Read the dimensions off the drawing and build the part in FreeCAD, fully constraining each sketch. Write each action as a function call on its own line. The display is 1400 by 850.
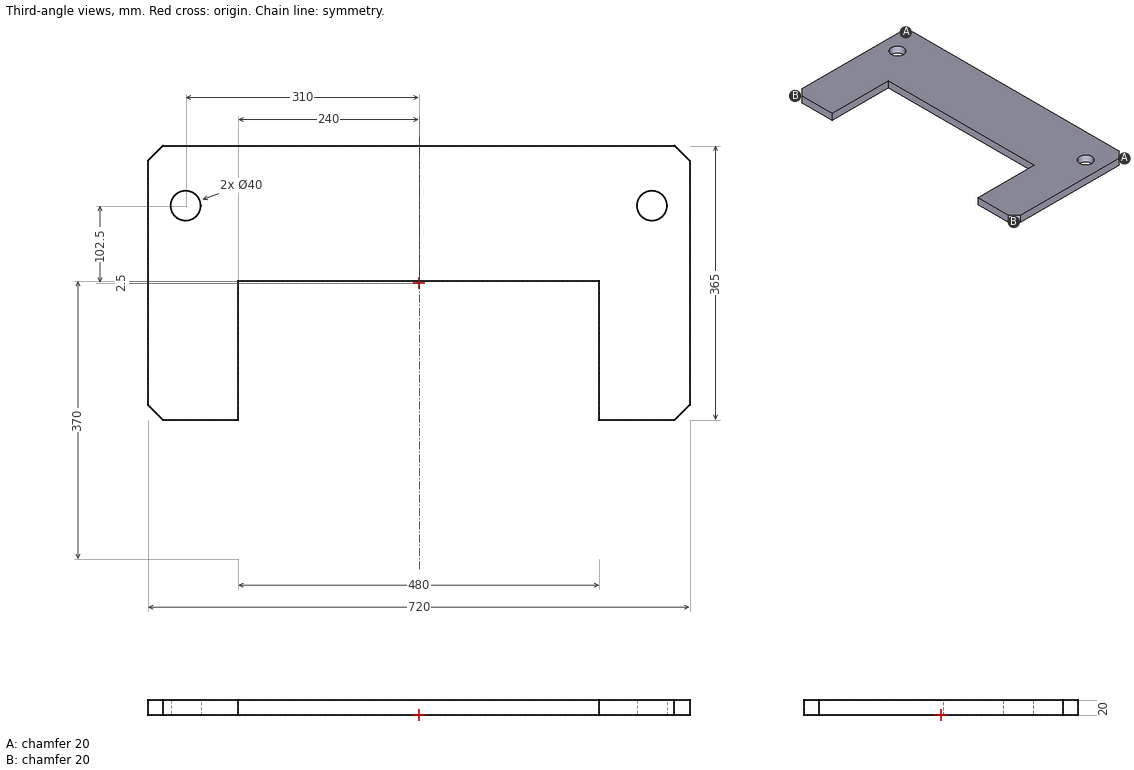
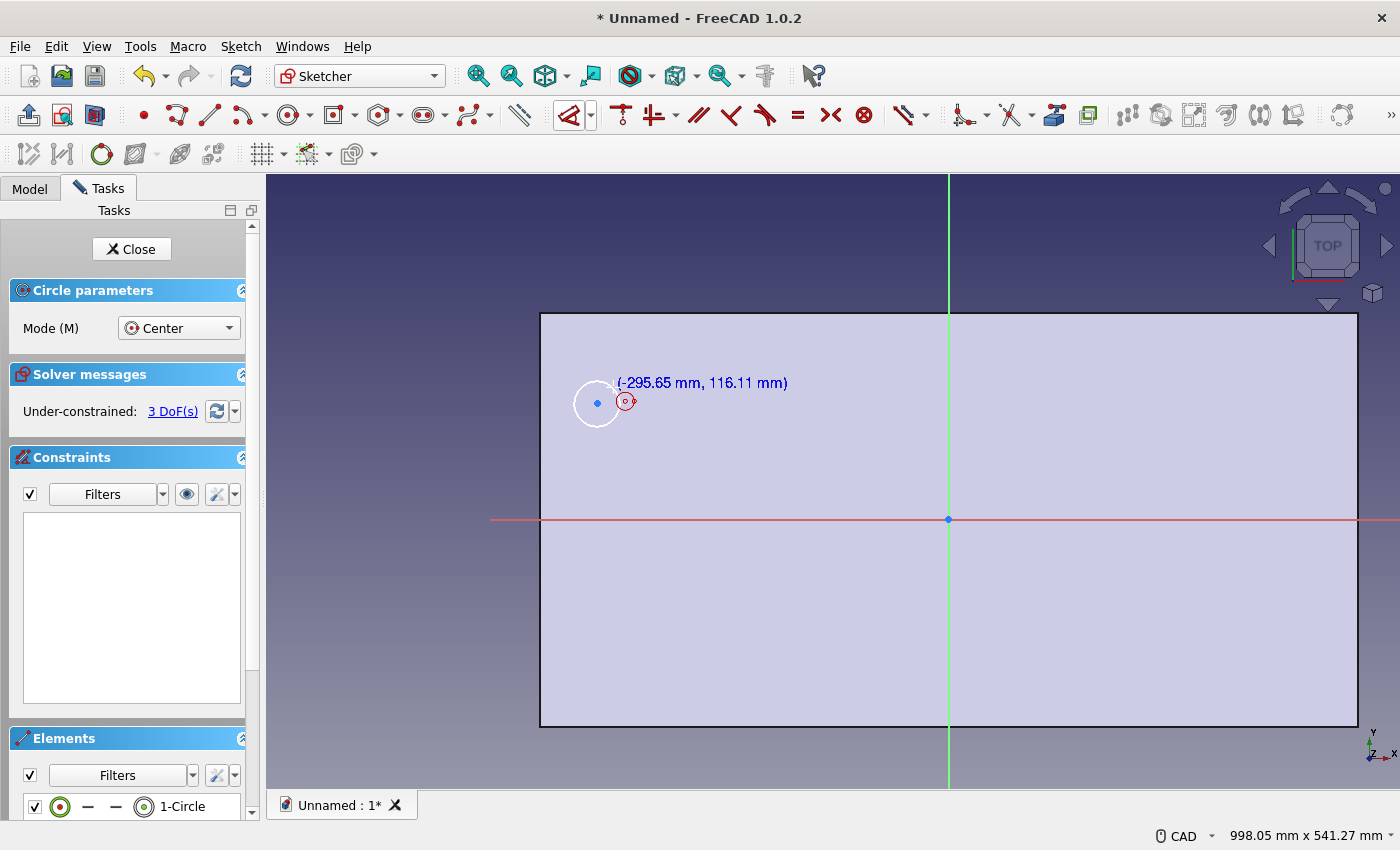
scroll(294, 622, down, 1)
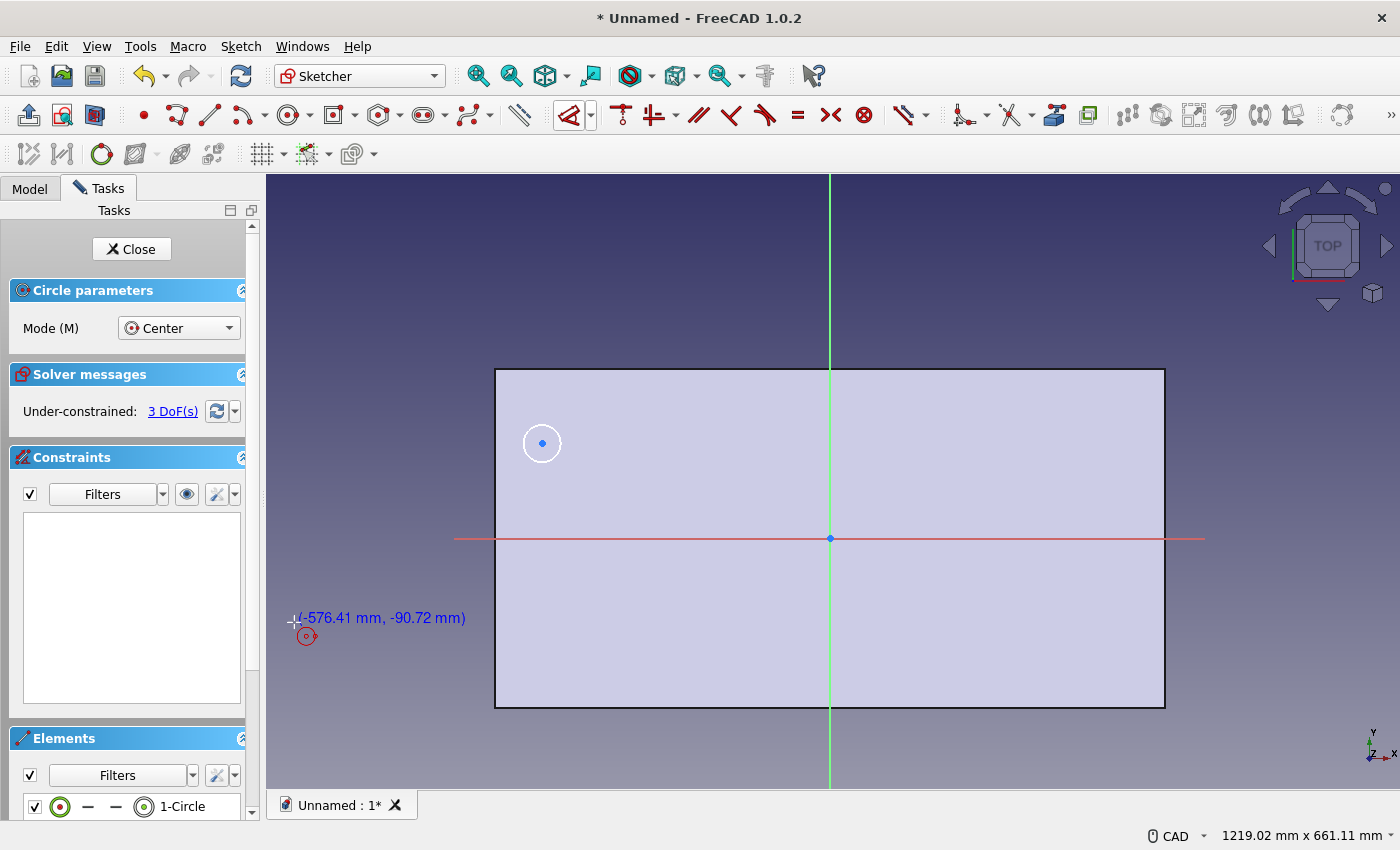
click(1119, 443)
click(1132, 430)
key(Escape)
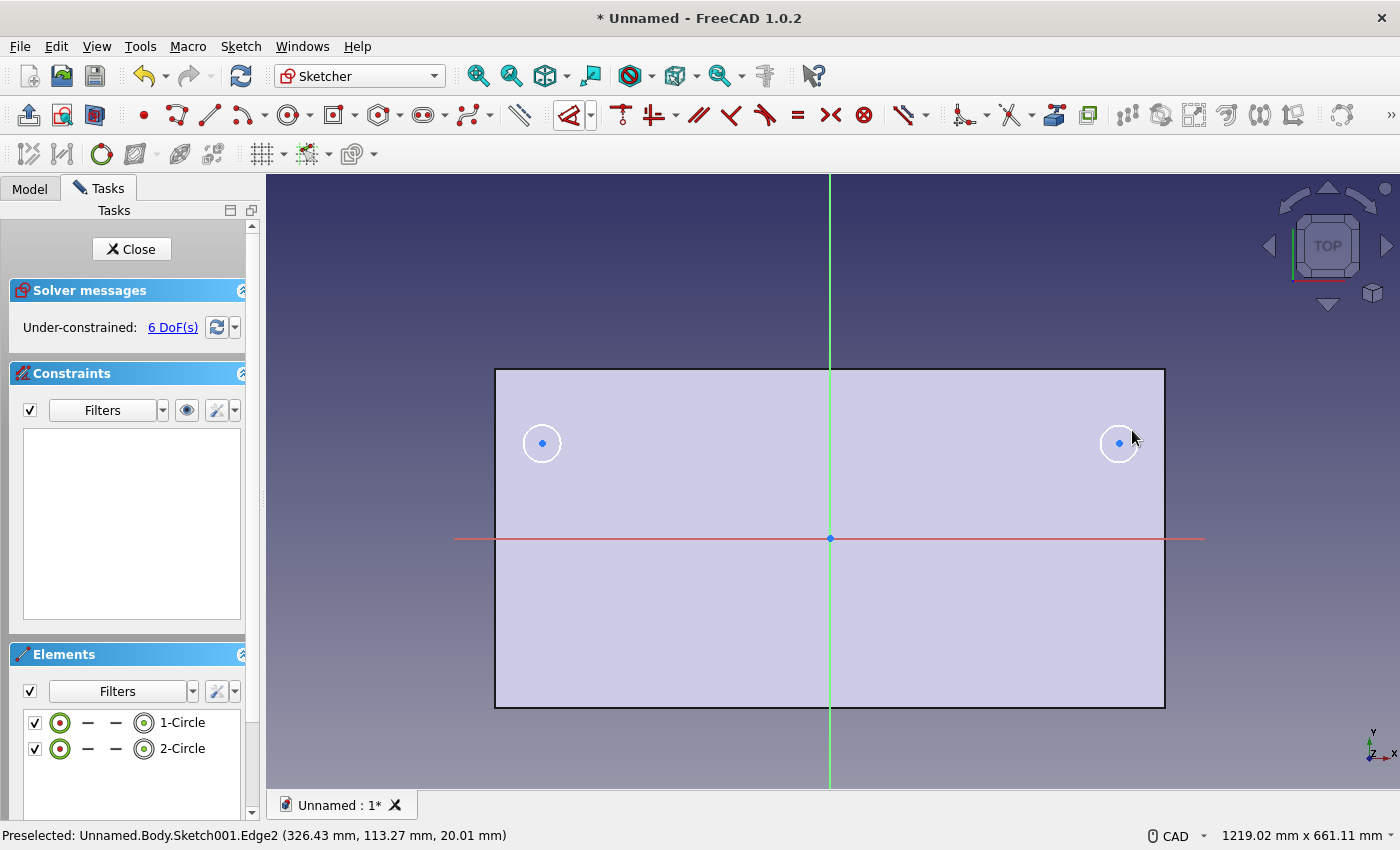
click(555, 431)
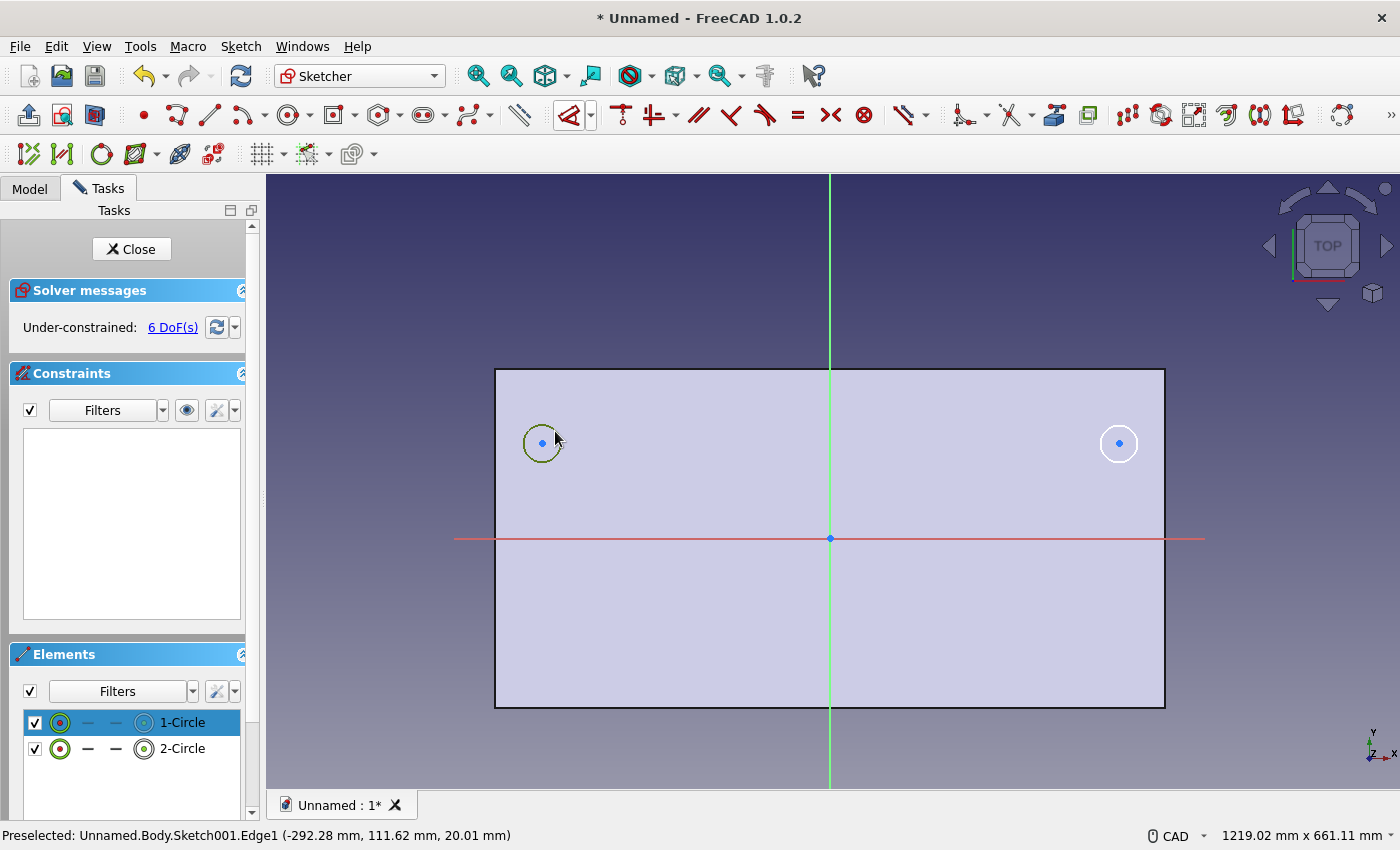
click(1132, 431)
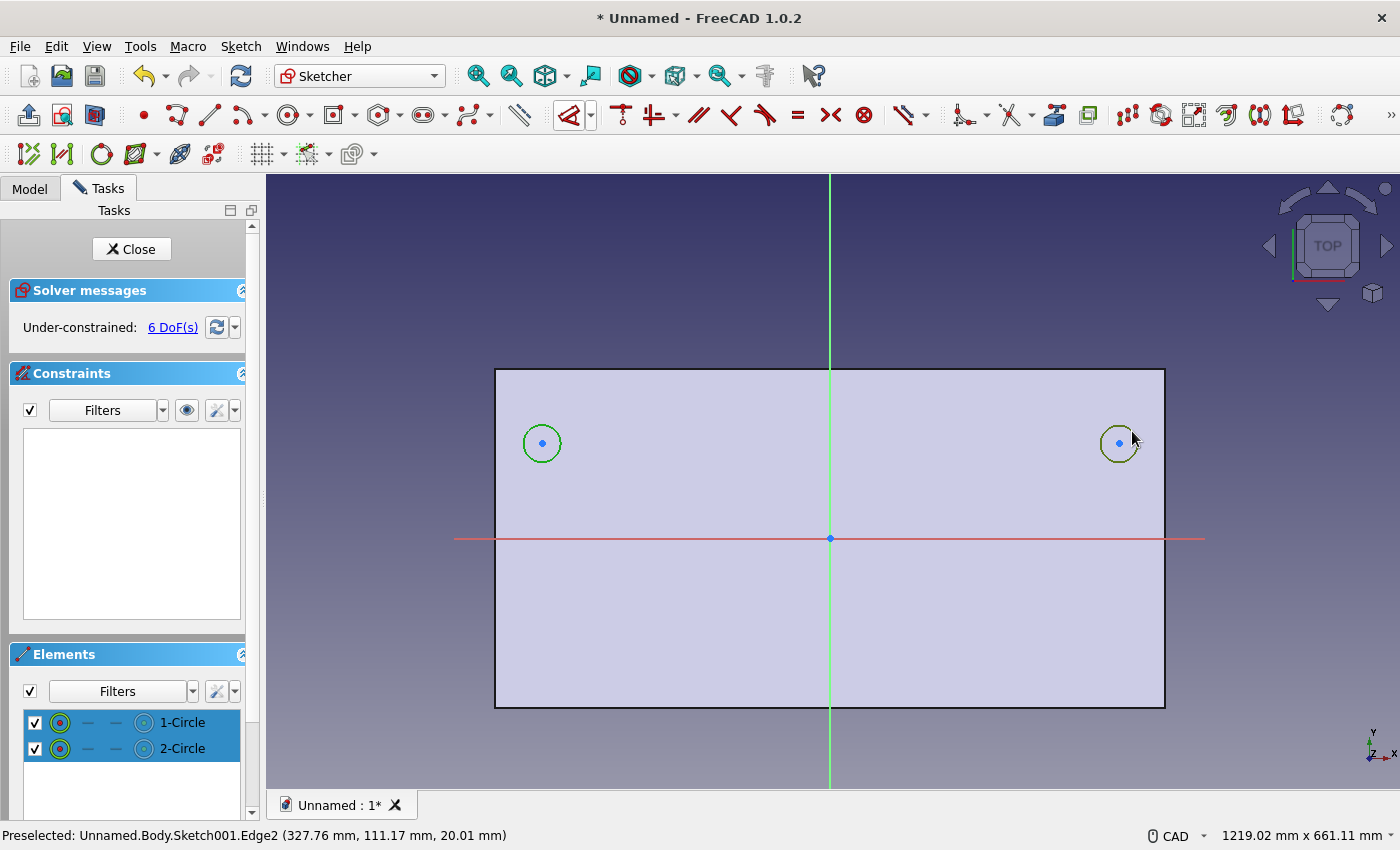
key(e)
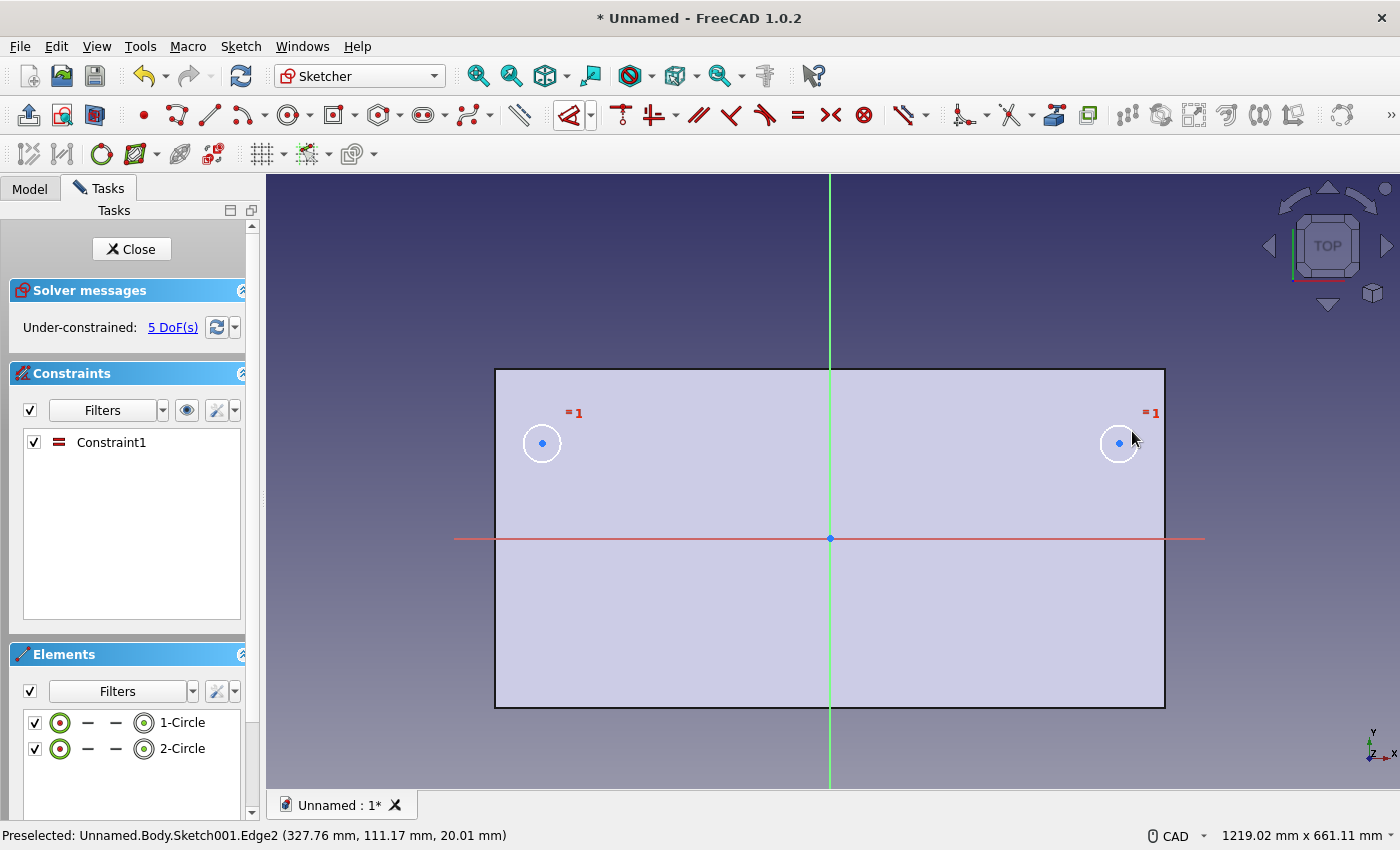
click(542, 444)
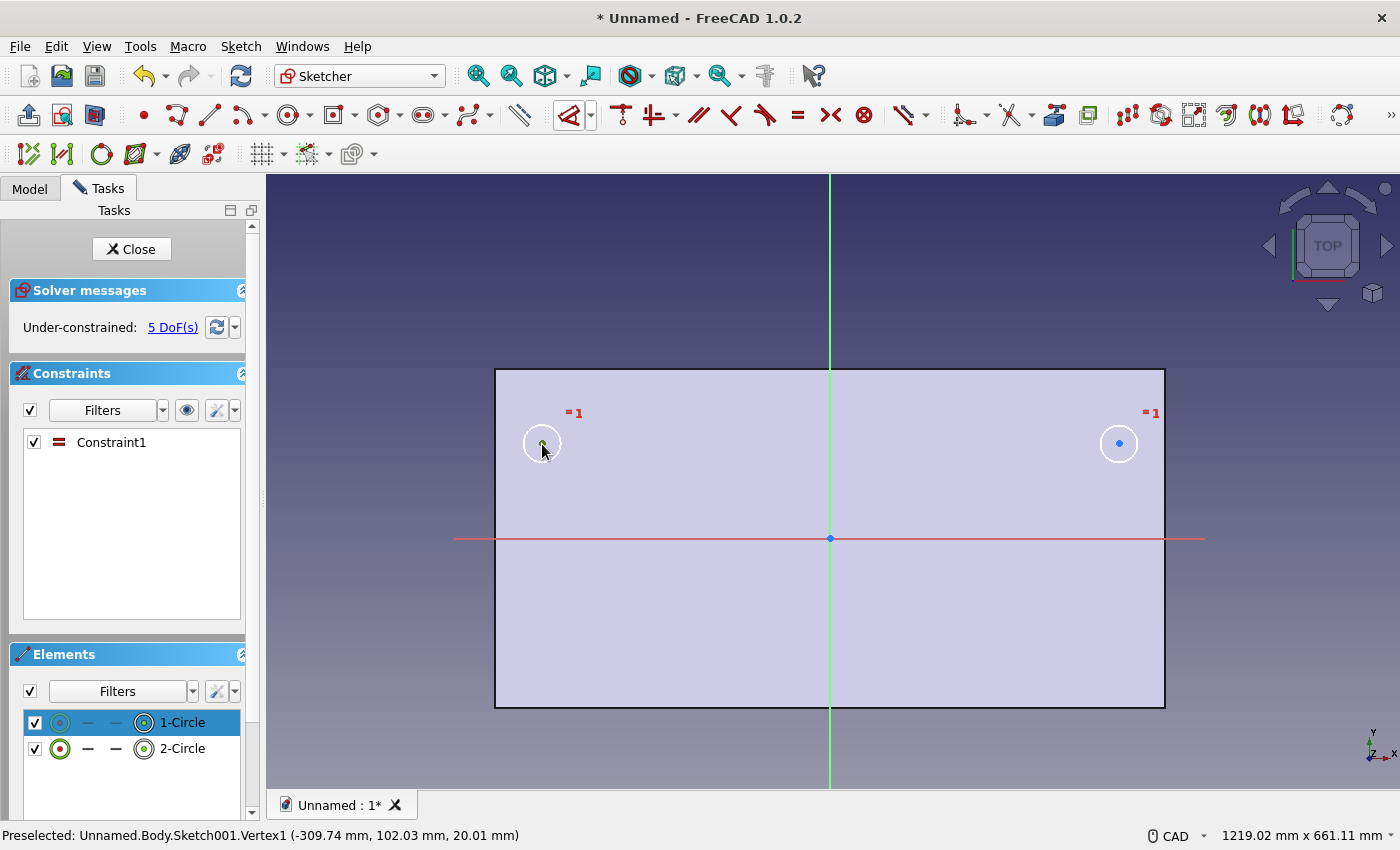
click(1119, 444)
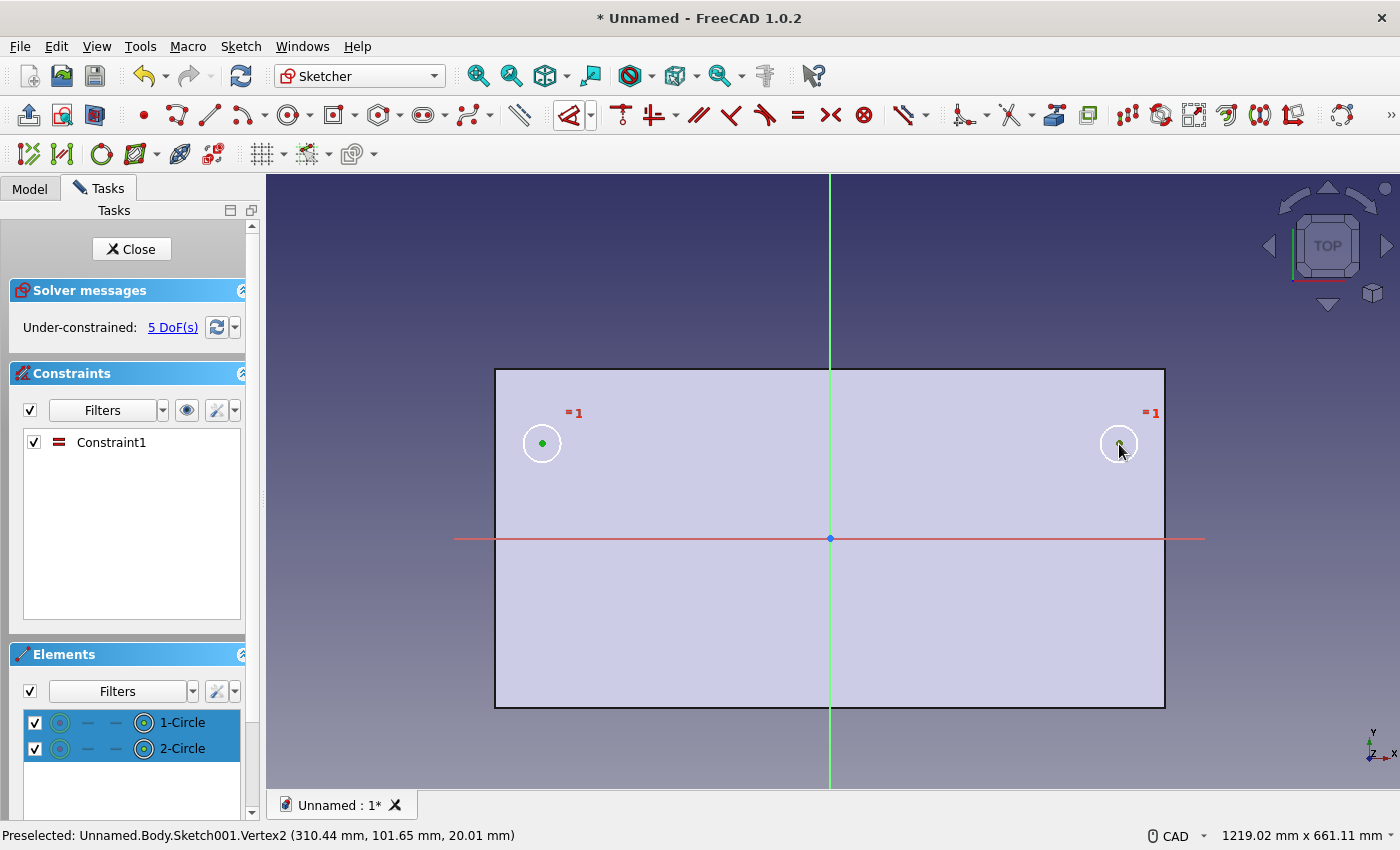
click(830, 721)